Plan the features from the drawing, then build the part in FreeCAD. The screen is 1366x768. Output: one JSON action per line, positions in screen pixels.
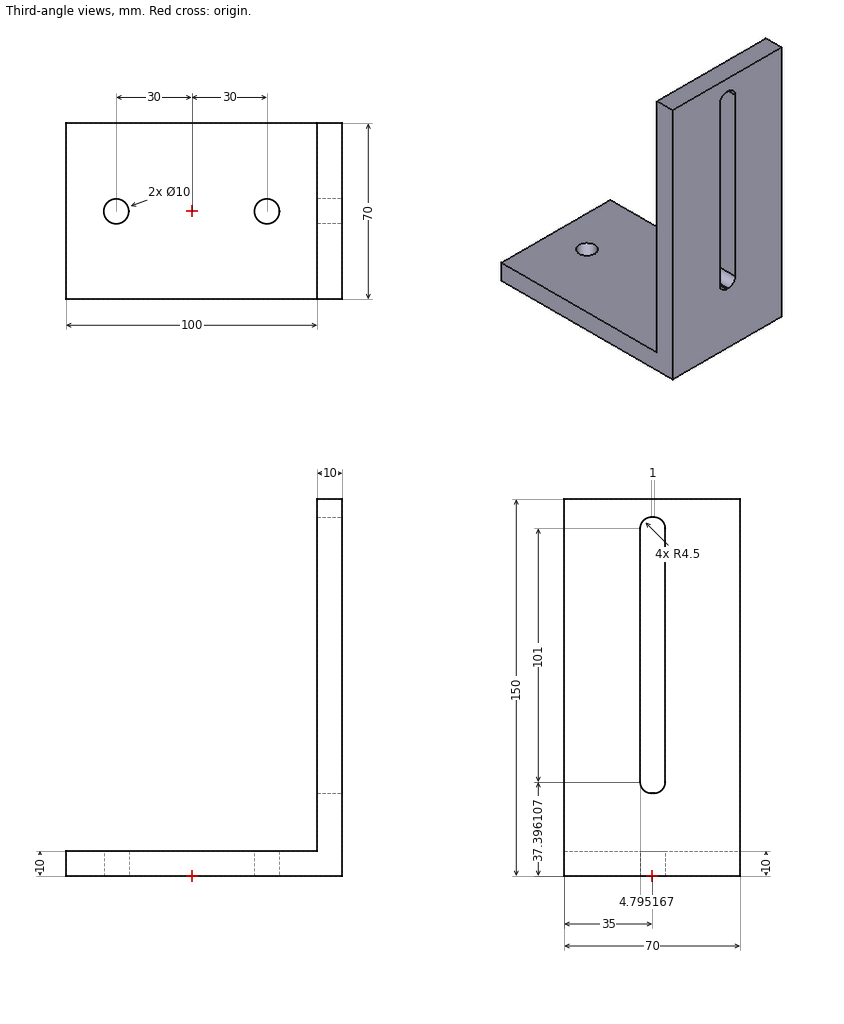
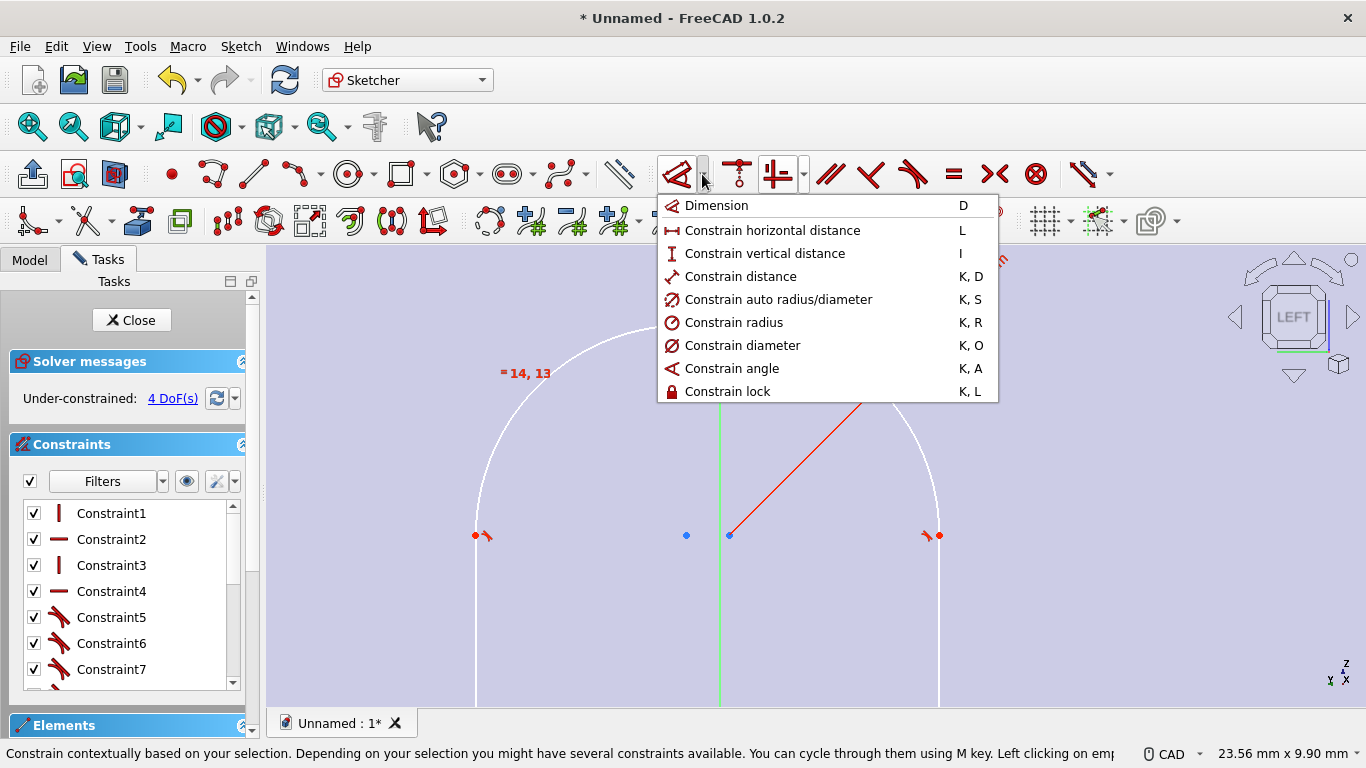
{"action": "left_click", "coordinate": [828, 230]}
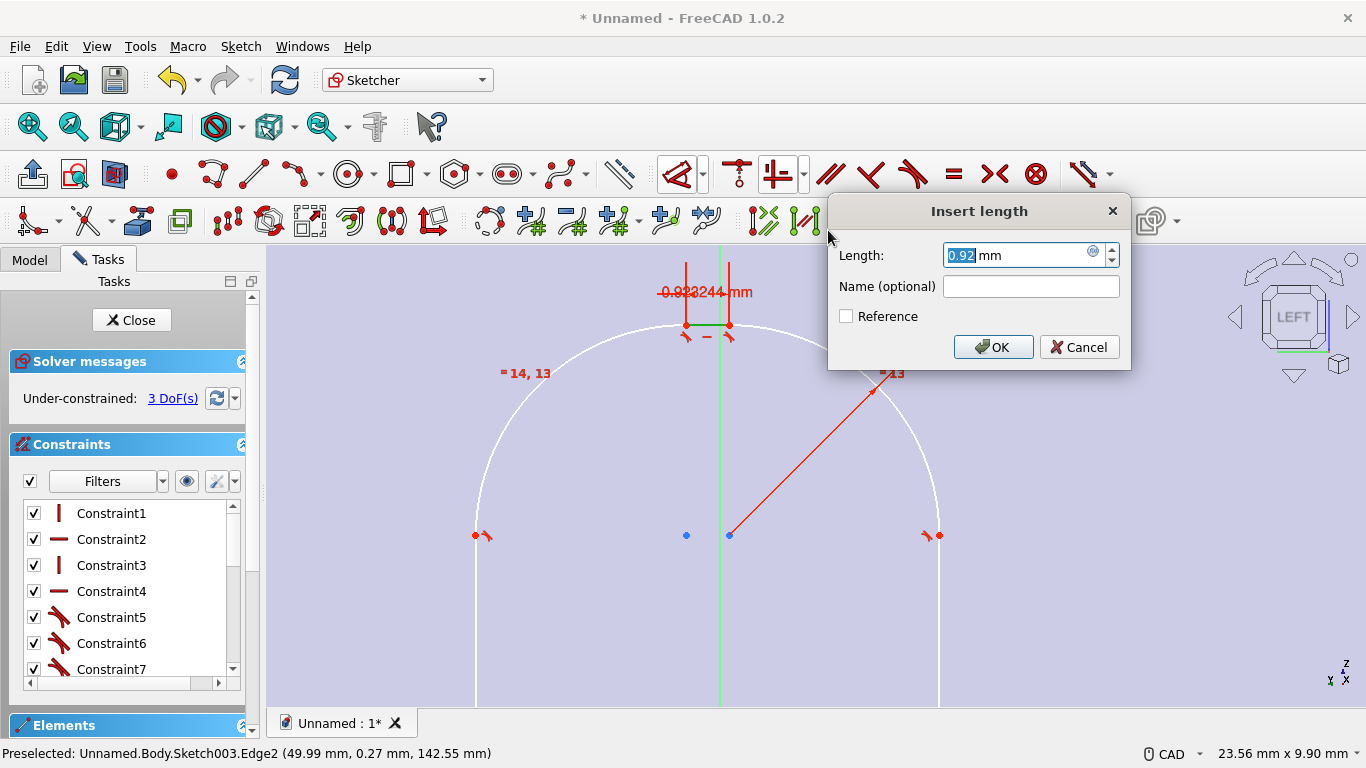
{"action": "type", "text": "1"}
{"action": "key", "text": "Return"}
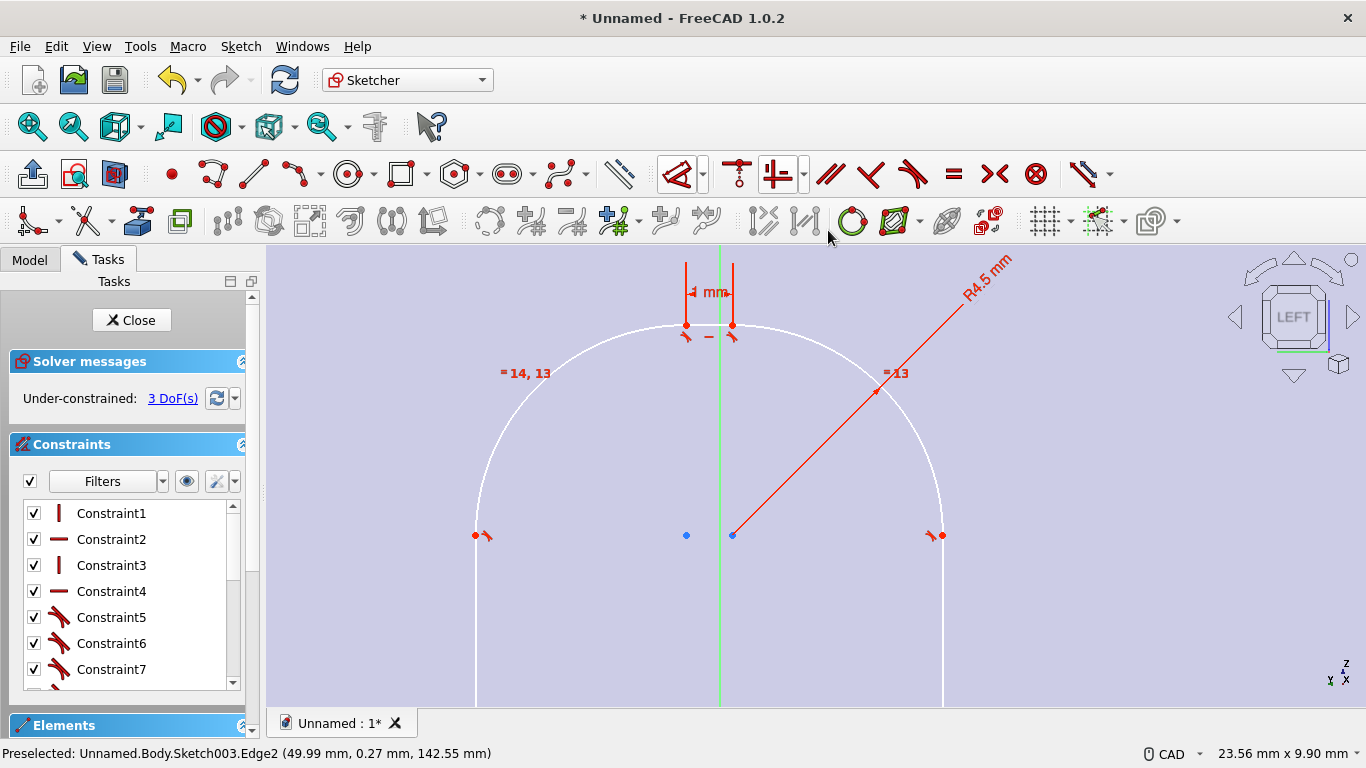
{"action": "scroll", "coordinate": [749, 310], "scroll_direction": "down", "scroll_amount": 15}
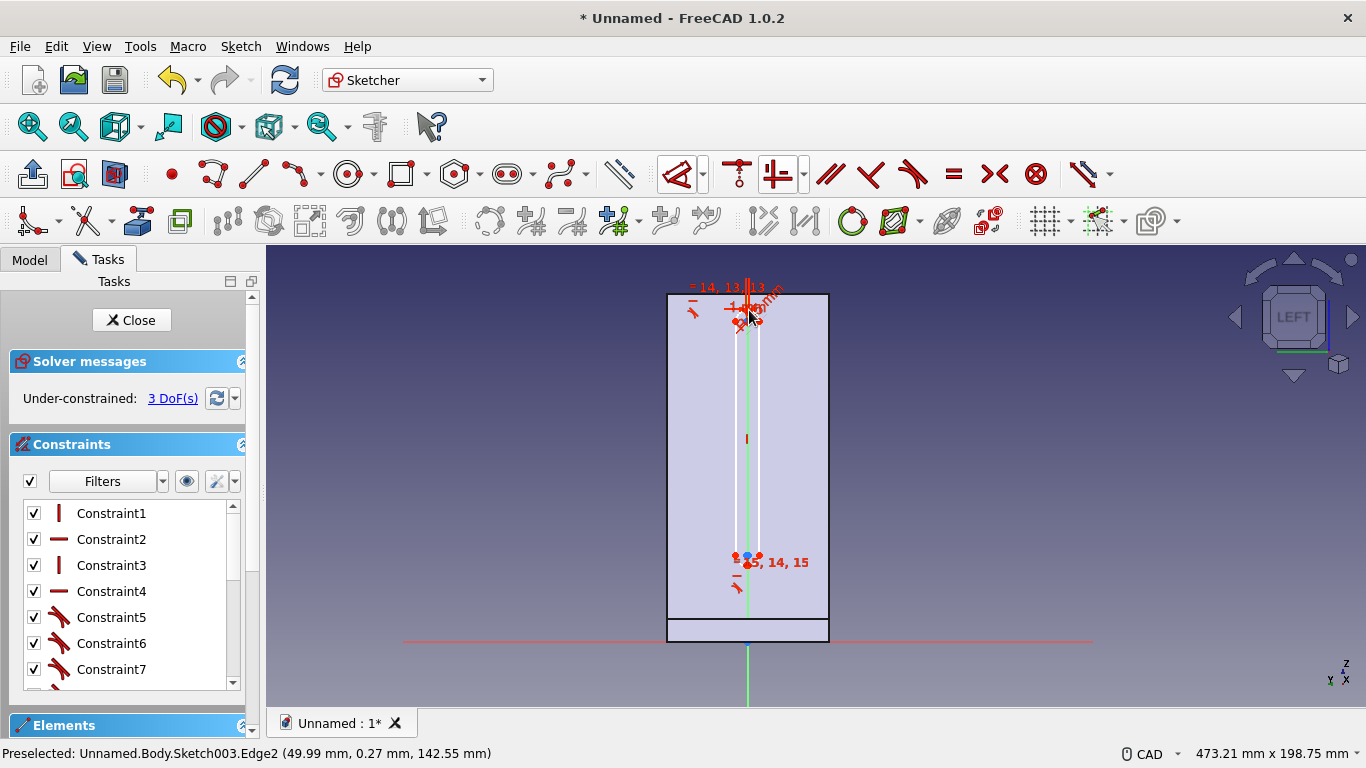
{"action": "scroll", "coordinate": [759, 485], "scroll_direction": "up", "scroll_amount": 2}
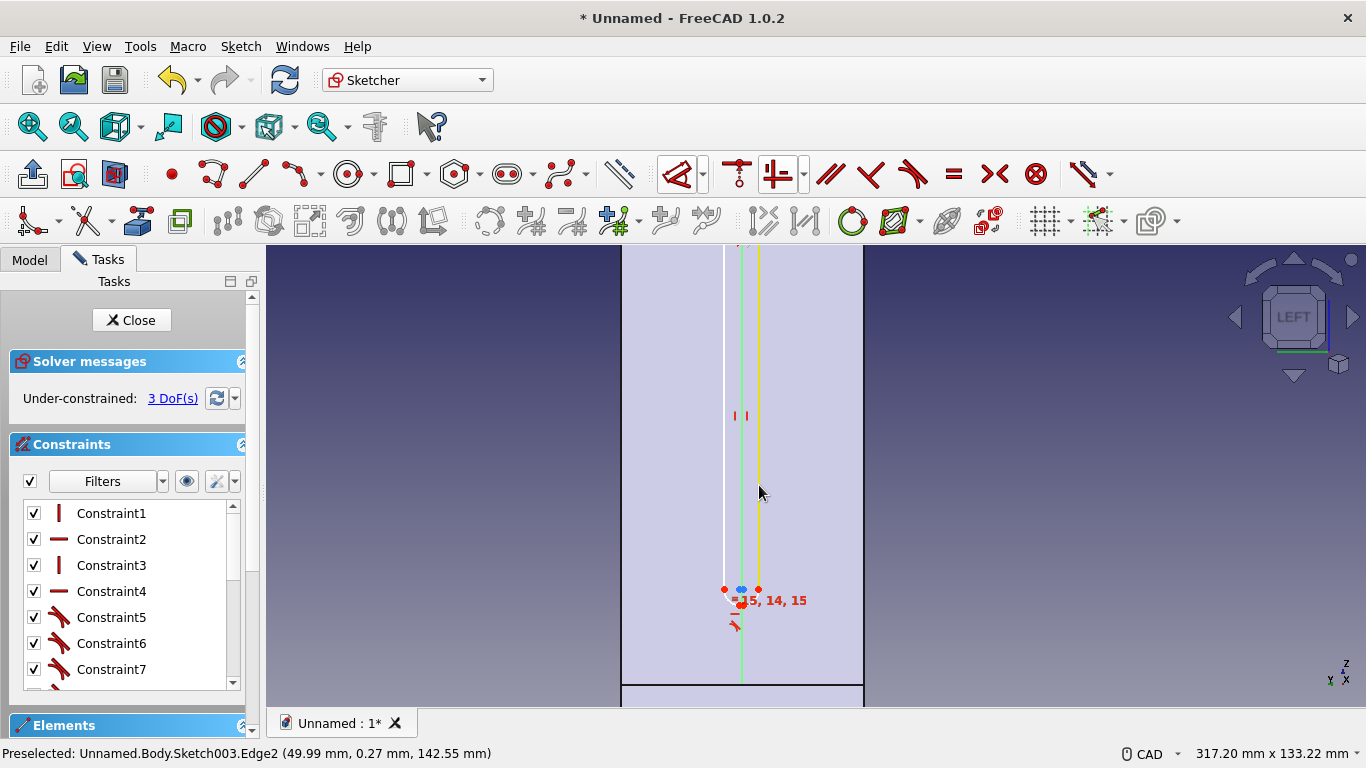
{"action": "left_click", "coordinate": [759, 485]}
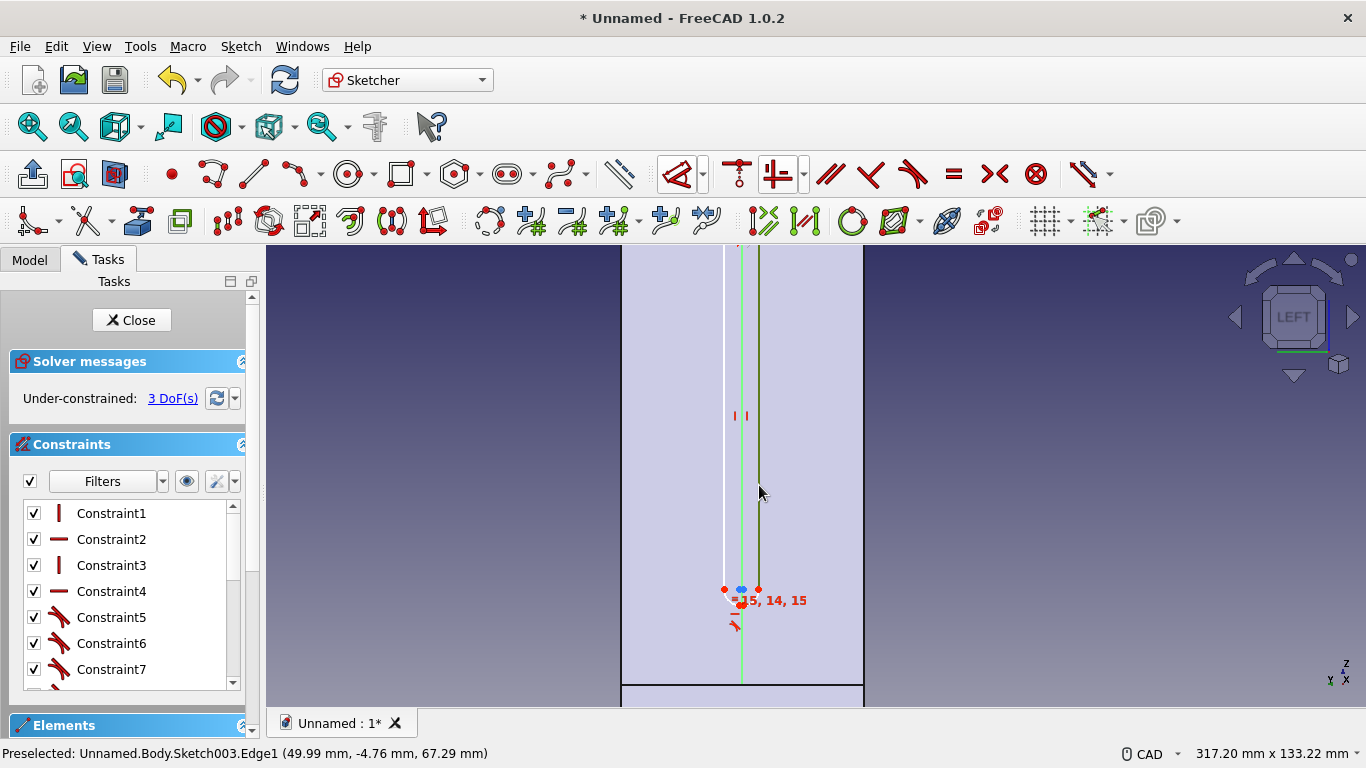
{"action": "left_click", "coordinate": [702, 174]}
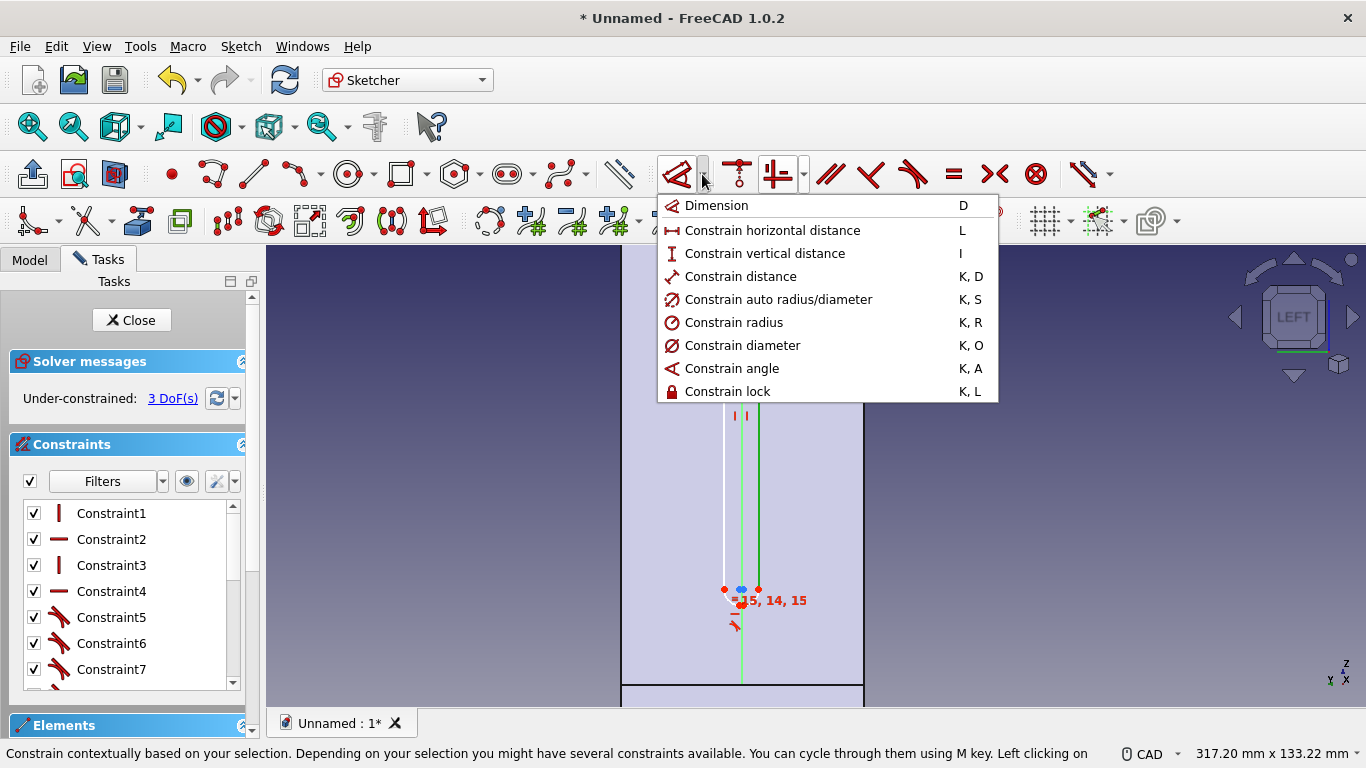
{"action": "left_click", "coordinate": [828, 254]}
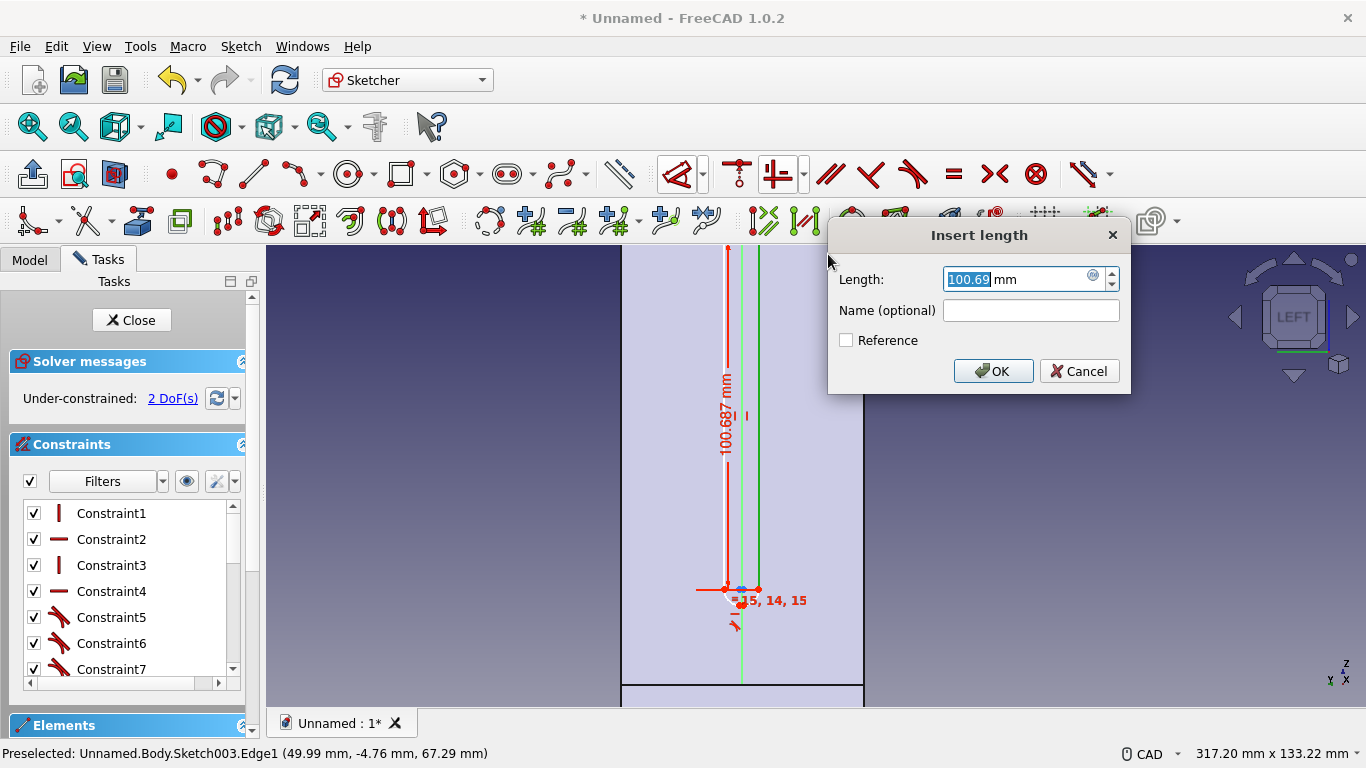
{"action": "type", "text": "101"}
{"action": "key", "text": "Return"}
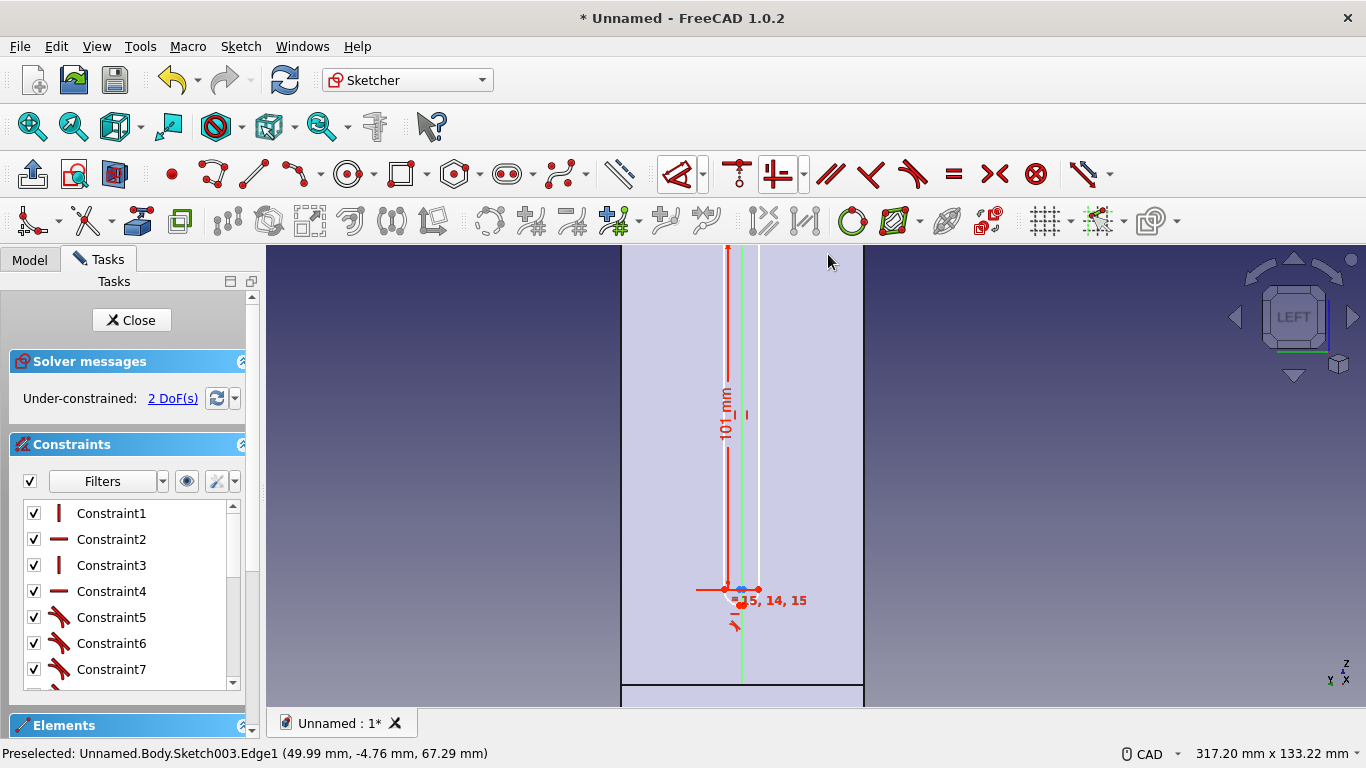
{"action": "scroll", "coordinate": [759, 590], "scroll_direction": "up", "scroll_amount": 5}